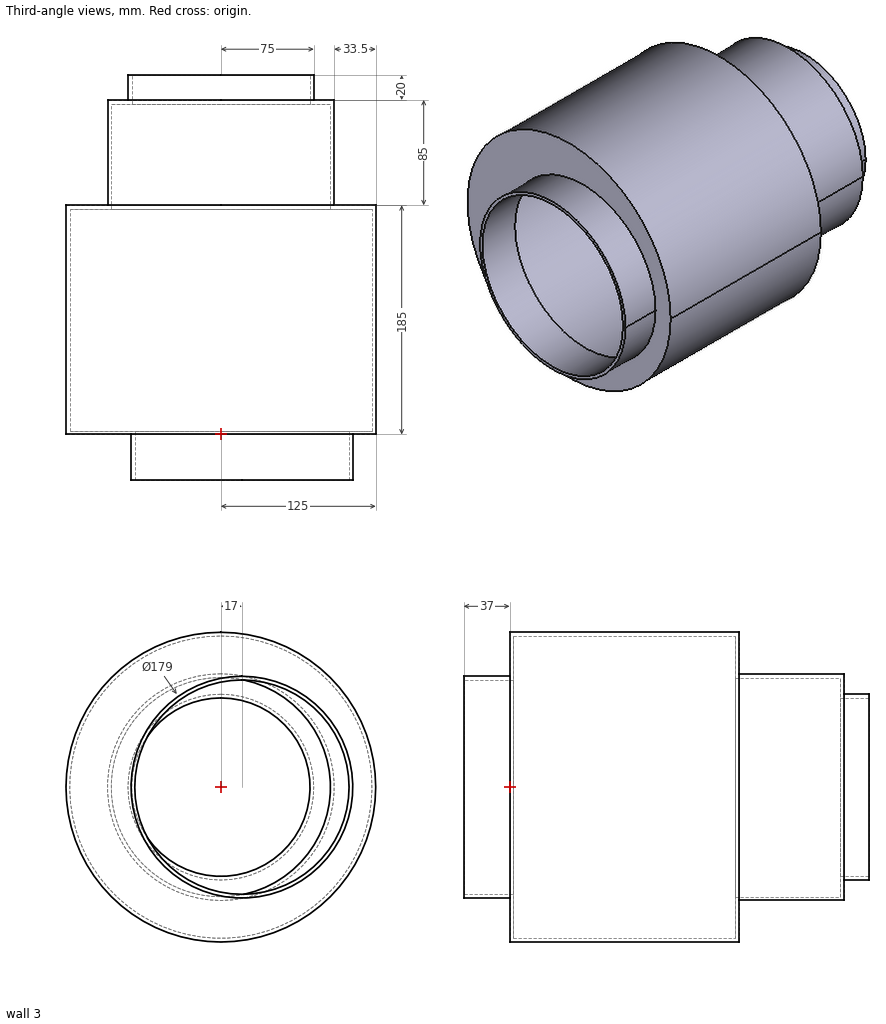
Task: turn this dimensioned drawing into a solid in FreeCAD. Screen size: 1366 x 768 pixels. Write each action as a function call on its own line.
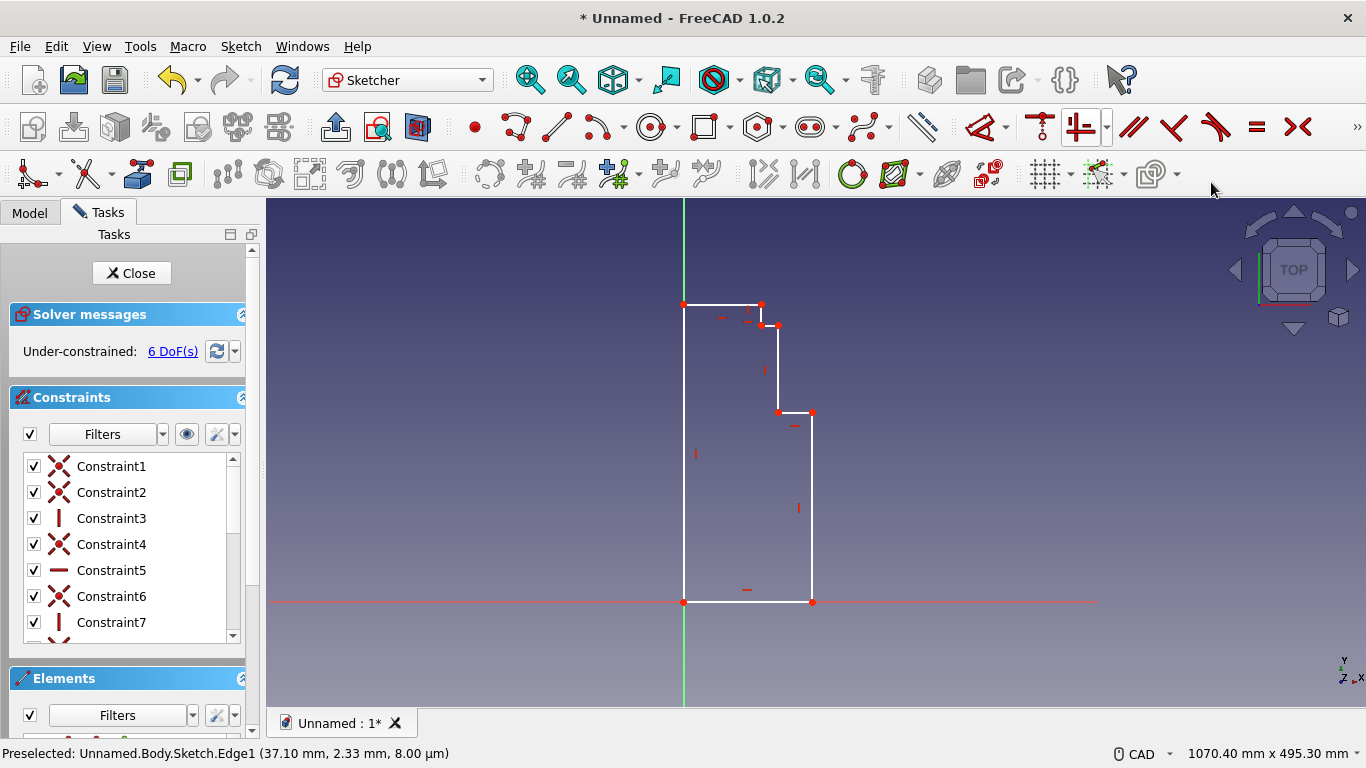
click(778, 387)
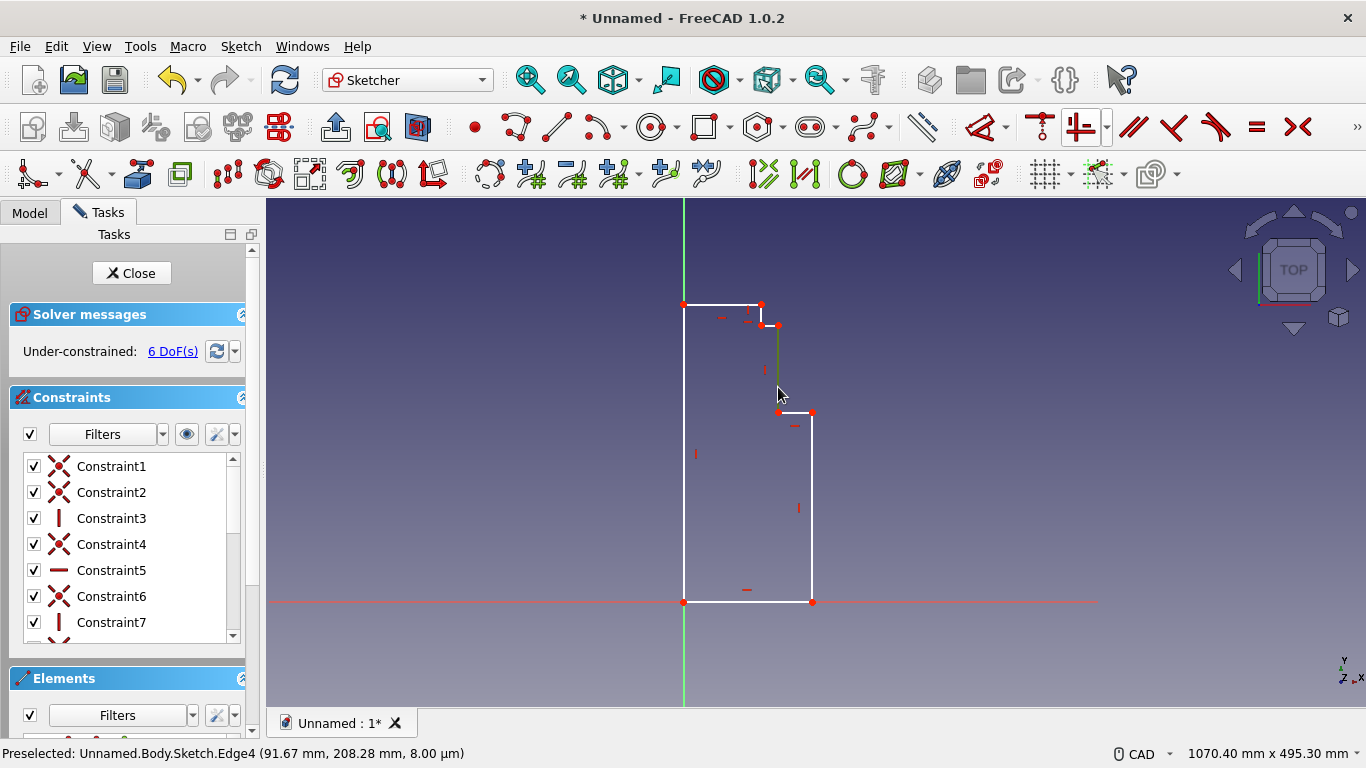
key(i)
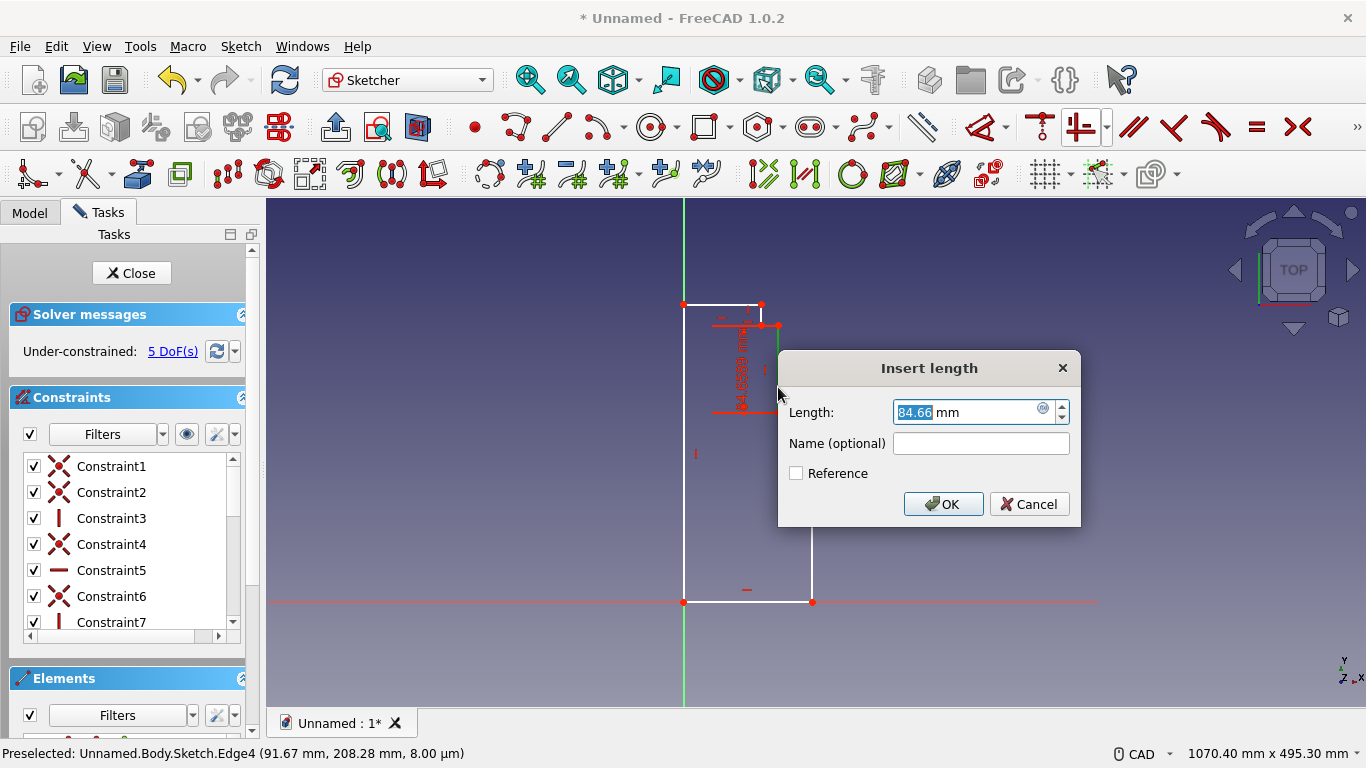
text(85)
key(Return)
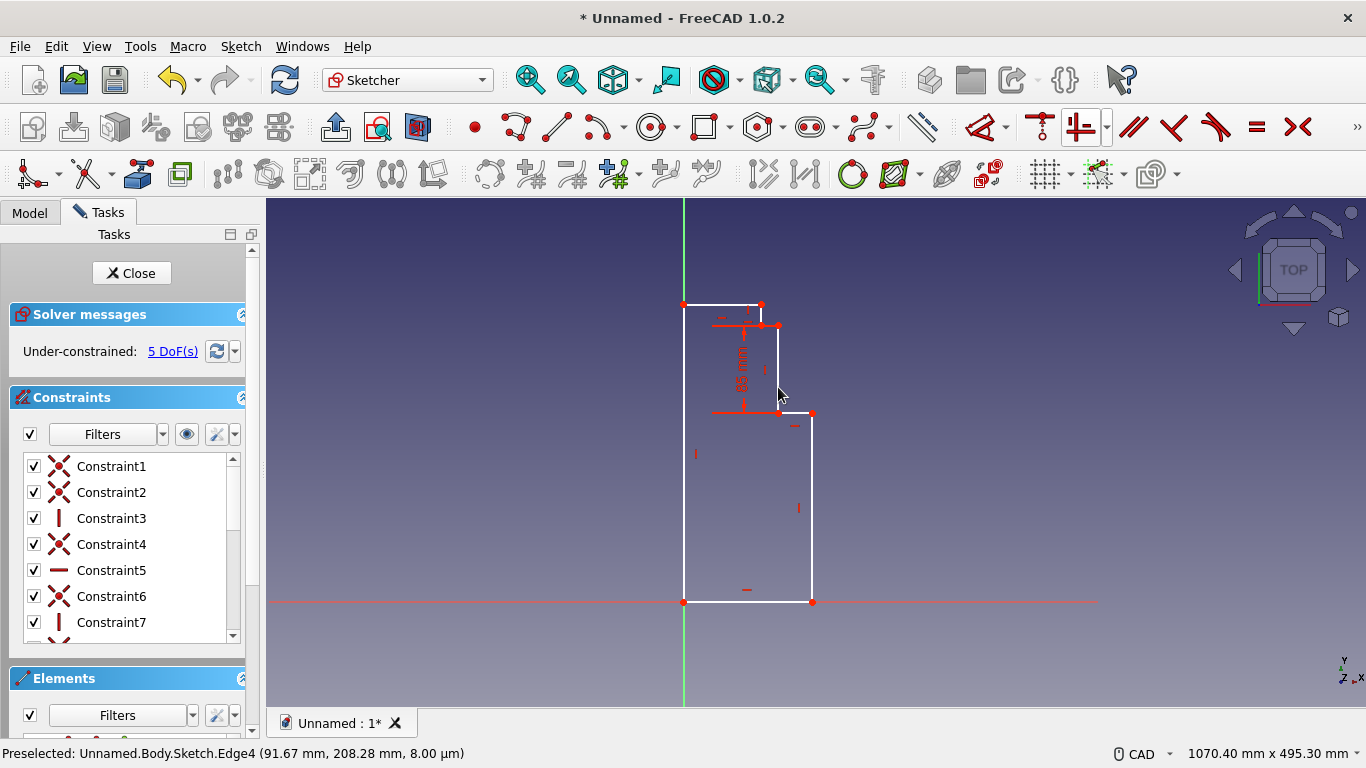
scroll(761, 315, up, 4)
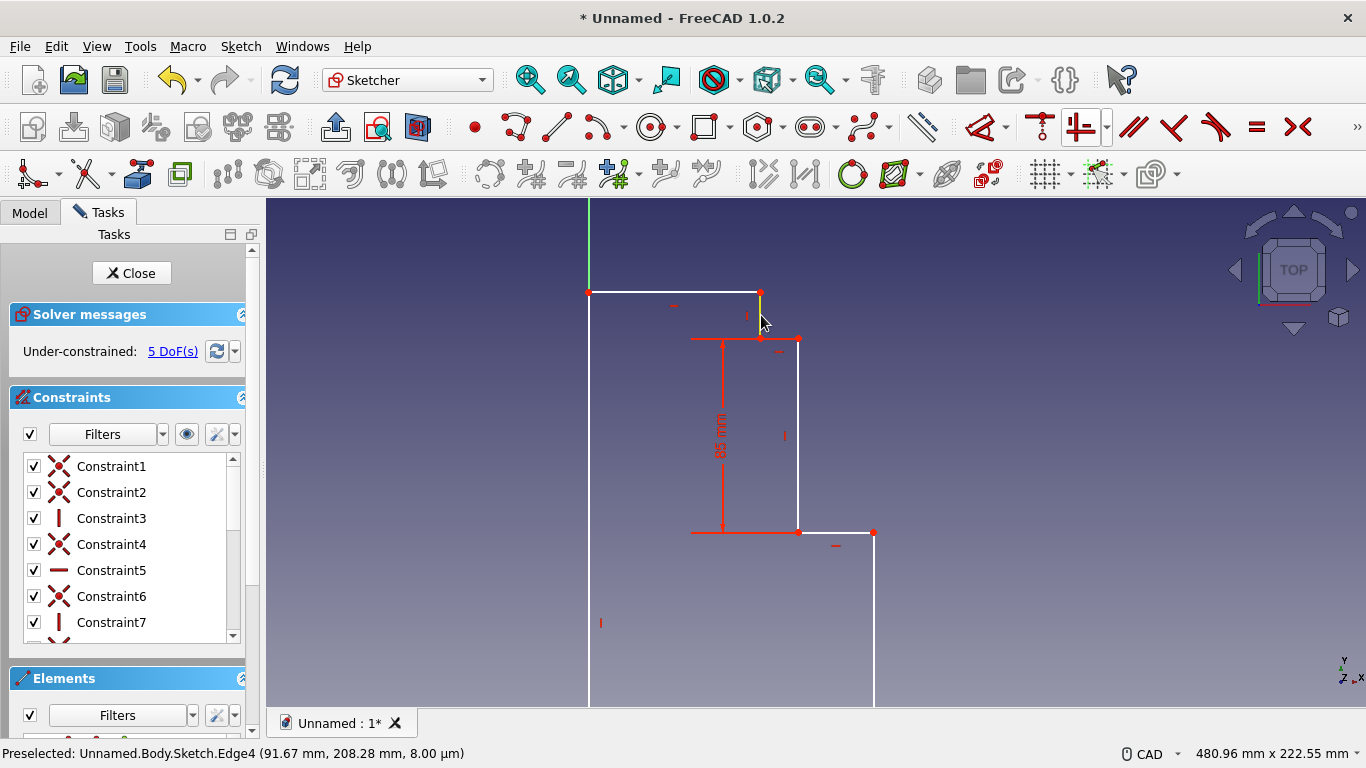
click(760, 316)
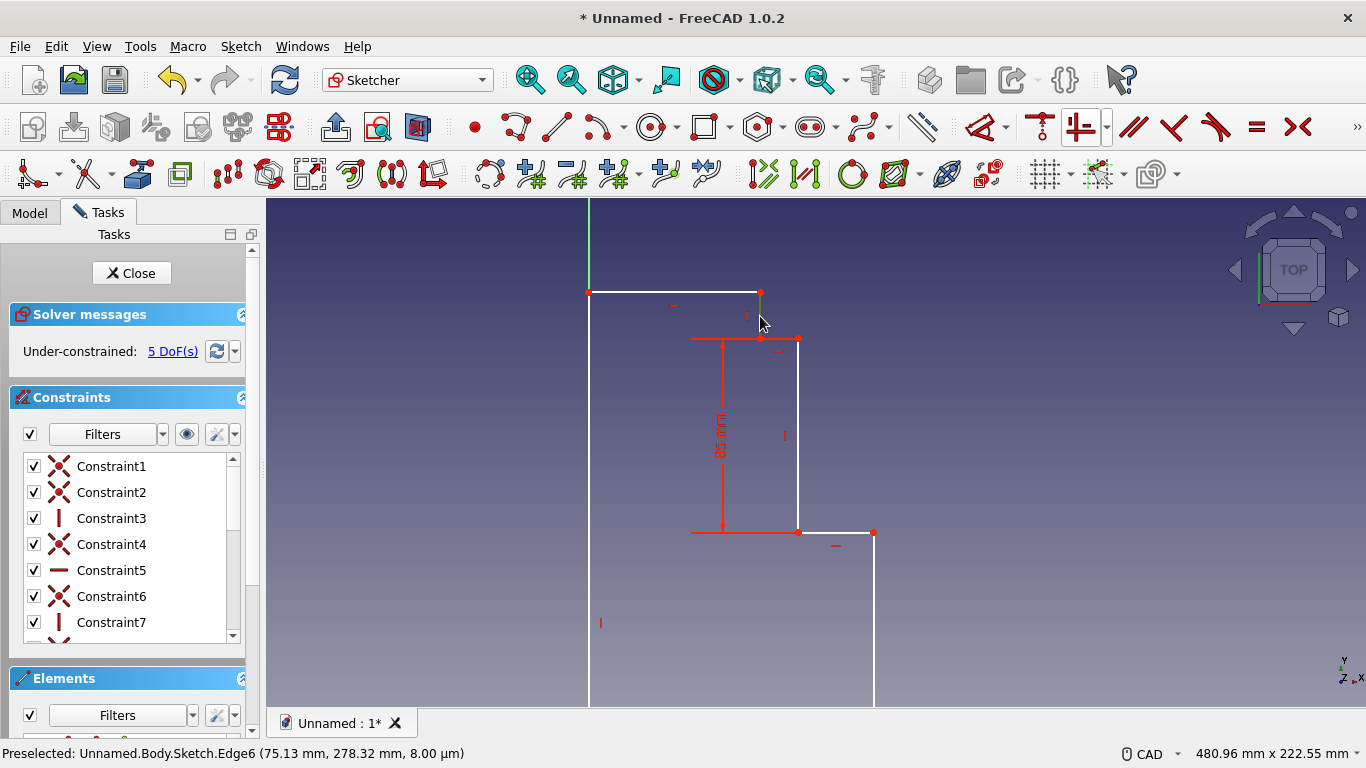
click(1006, 128)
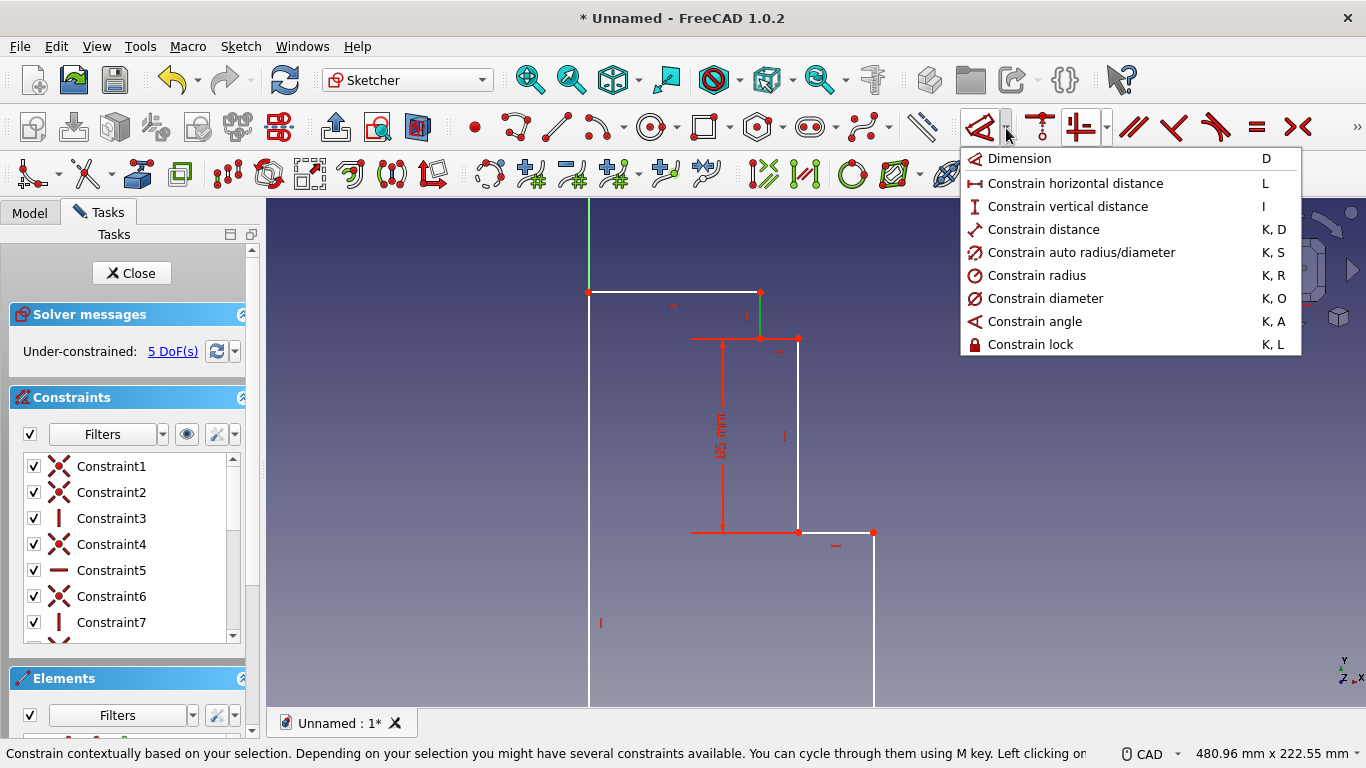
click(1131, 206)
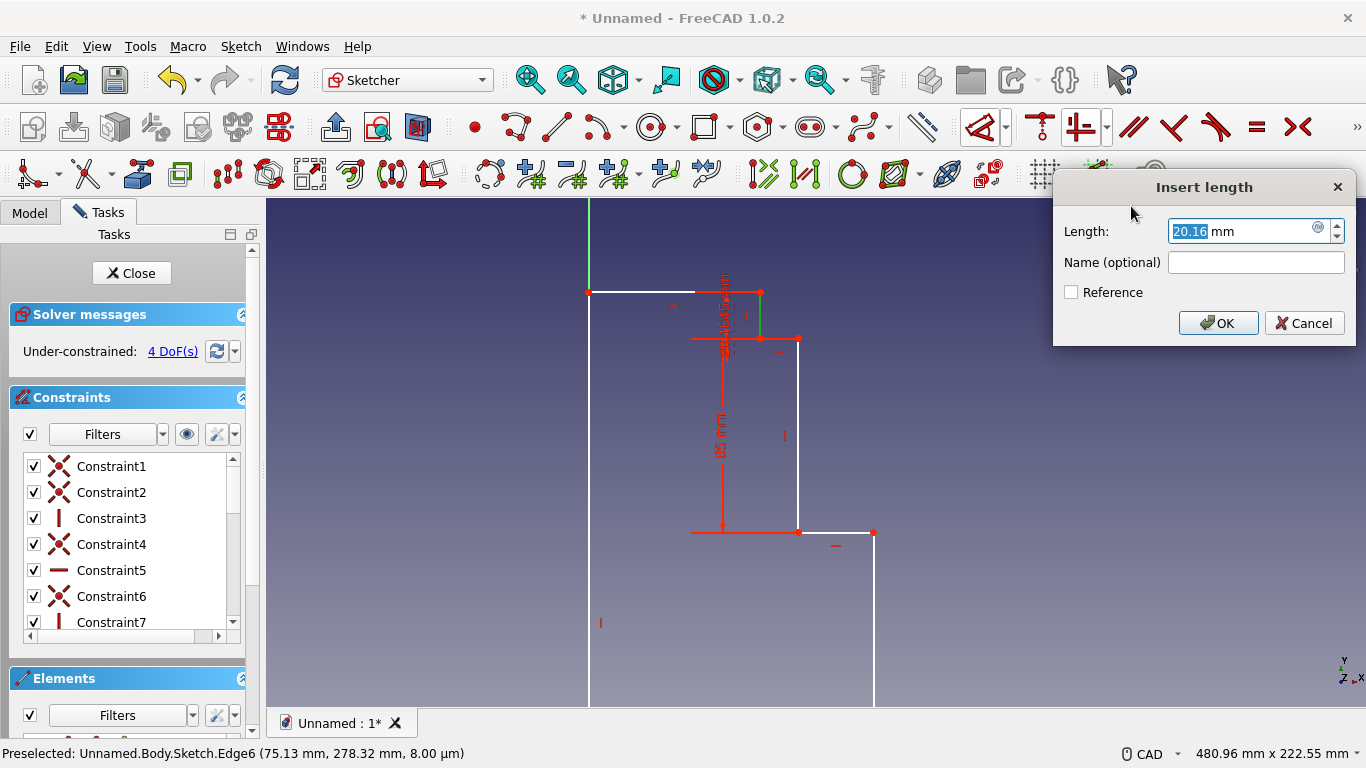
text(20)
key(Return)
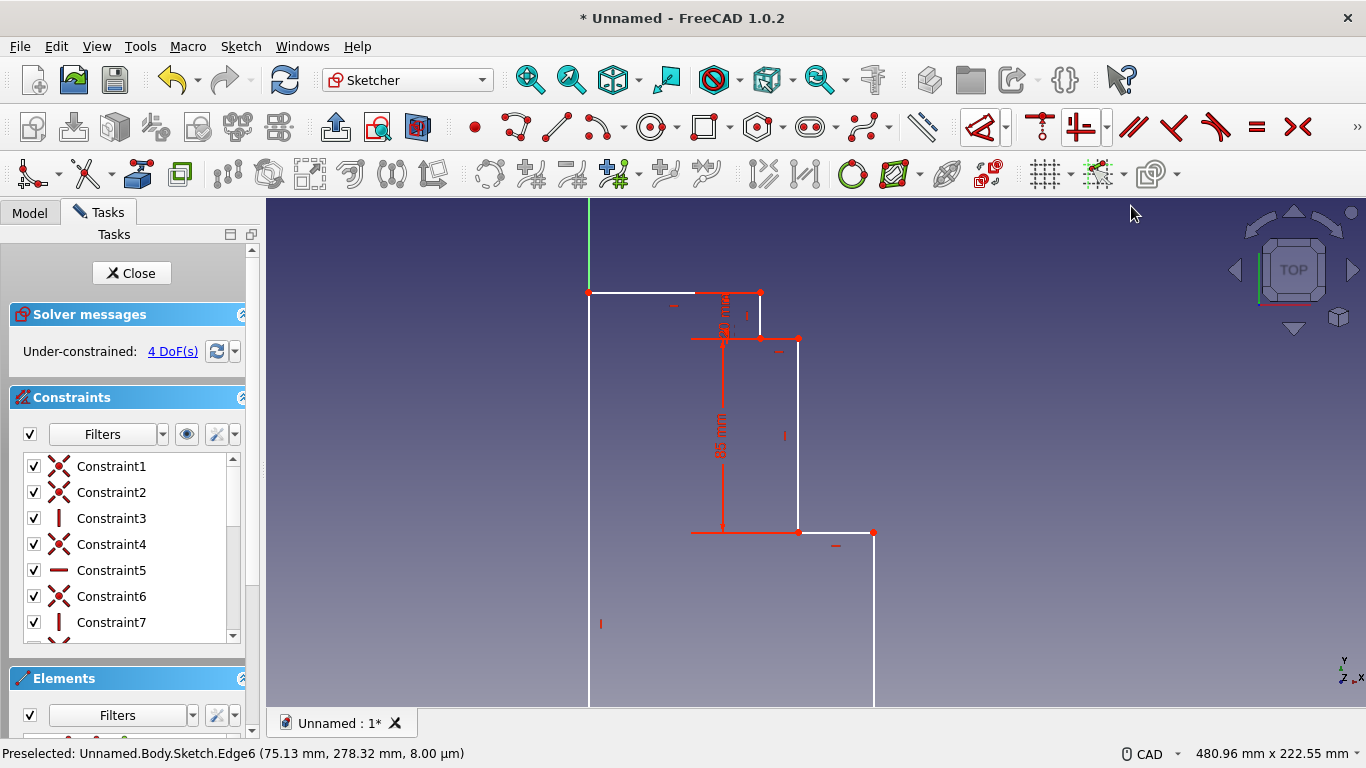
click(709, 293)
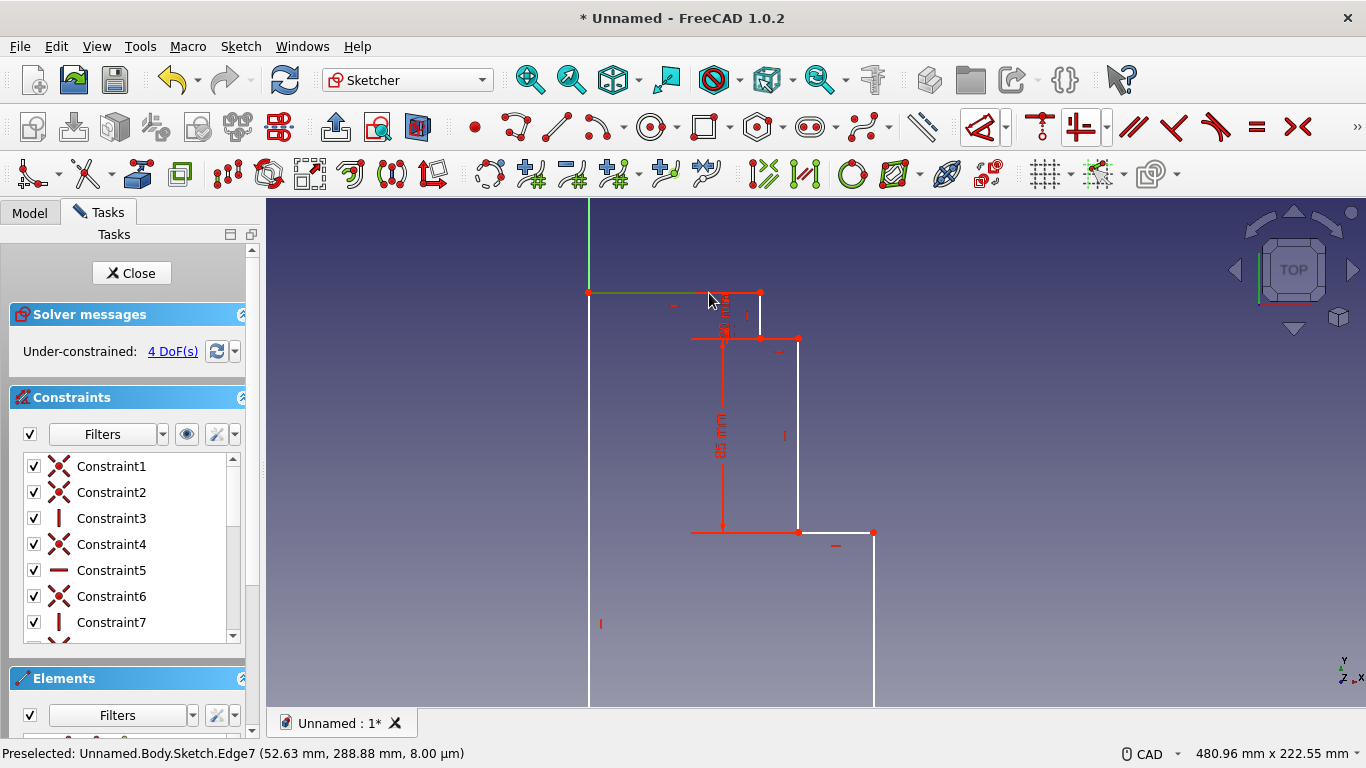
click(1006, 128)